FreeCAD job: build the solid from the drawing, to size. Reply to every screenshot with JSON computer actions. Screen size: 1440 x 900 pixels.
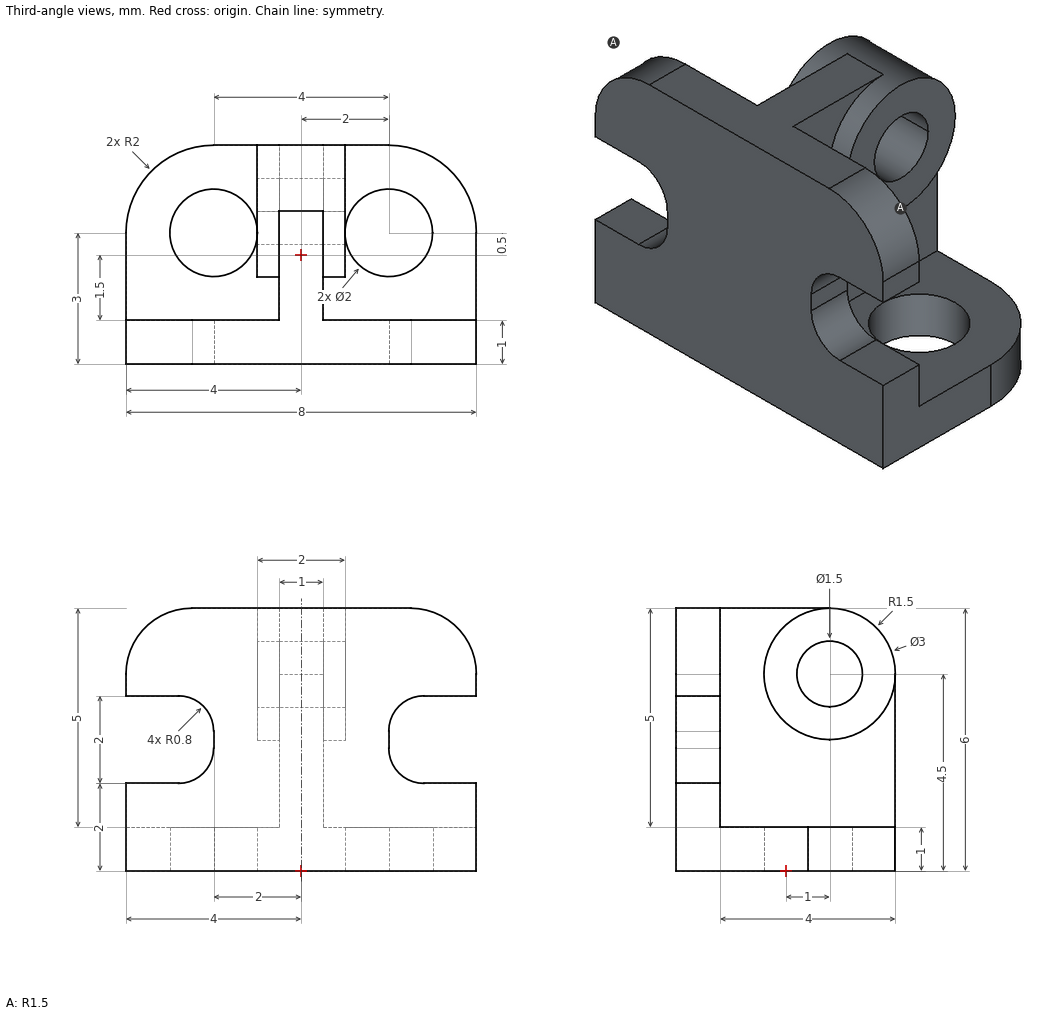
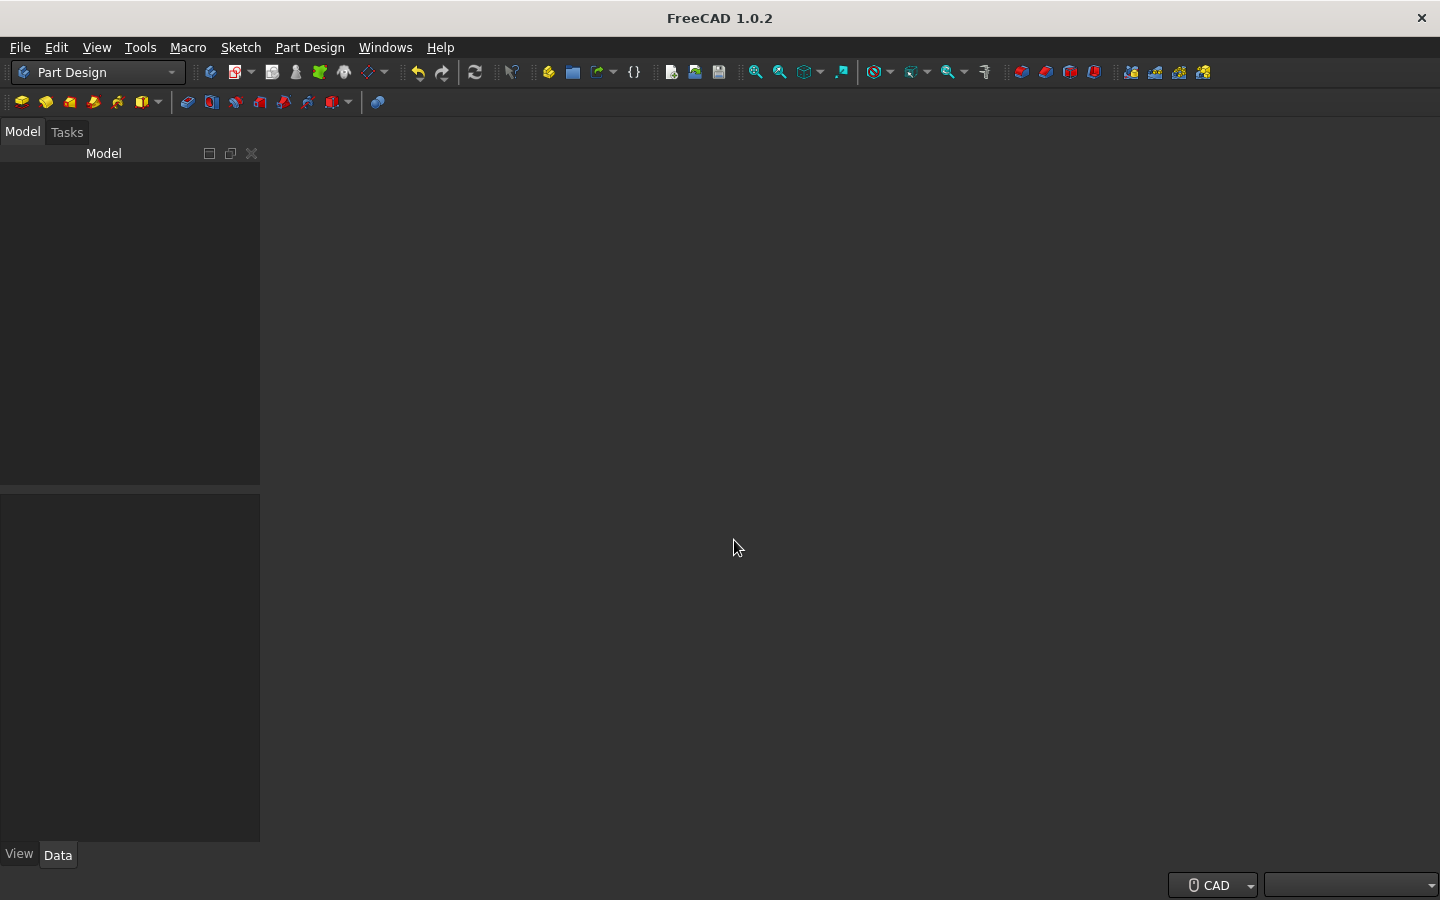
{"action": "left_click", "coordinate": [672, 72]}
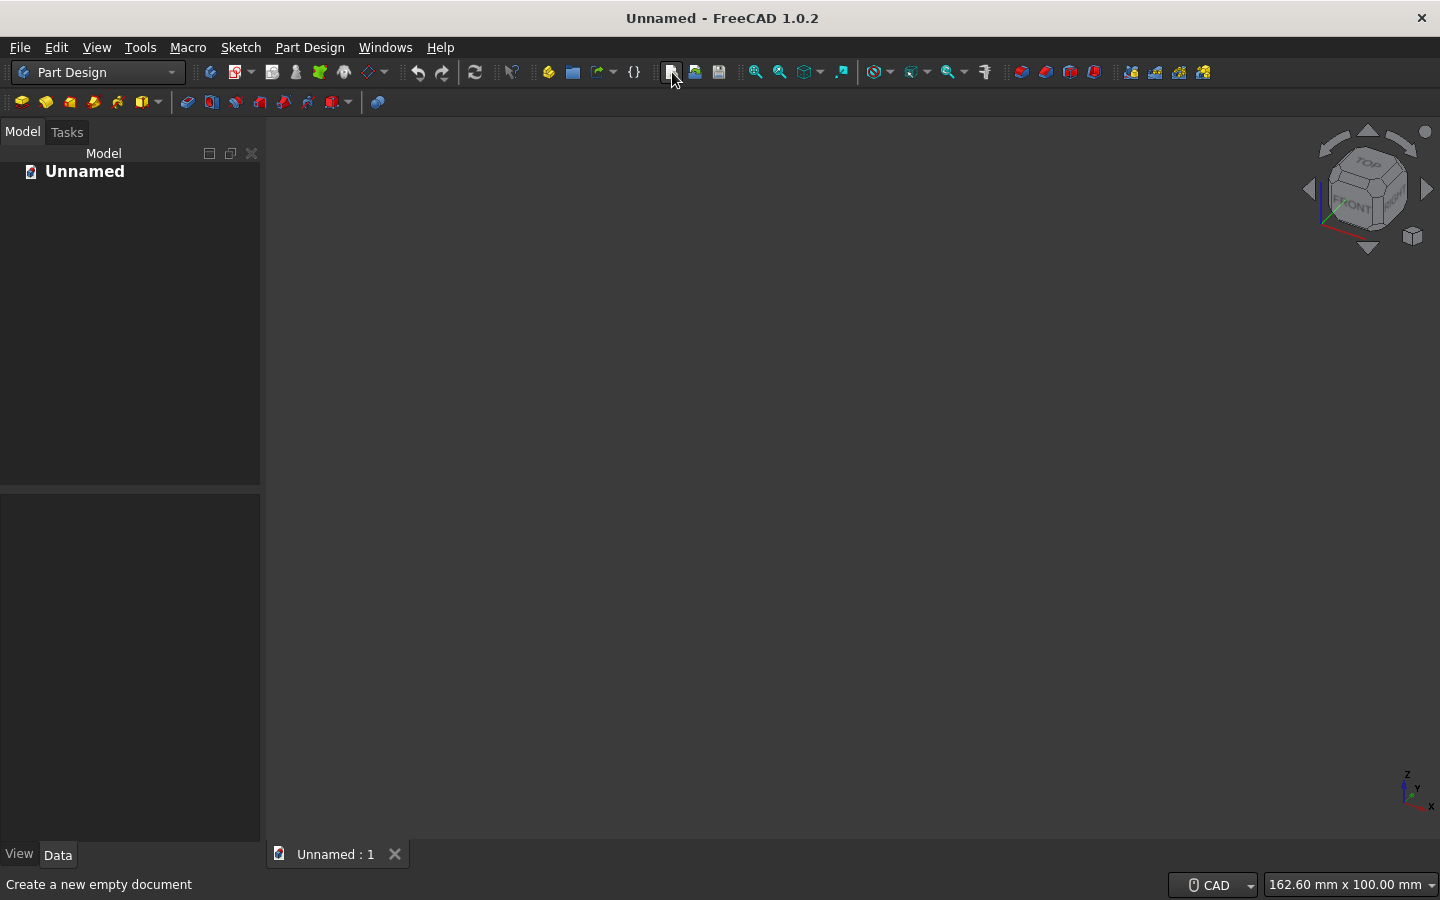
{"action": "left_click", "coordinate": [236, 72]}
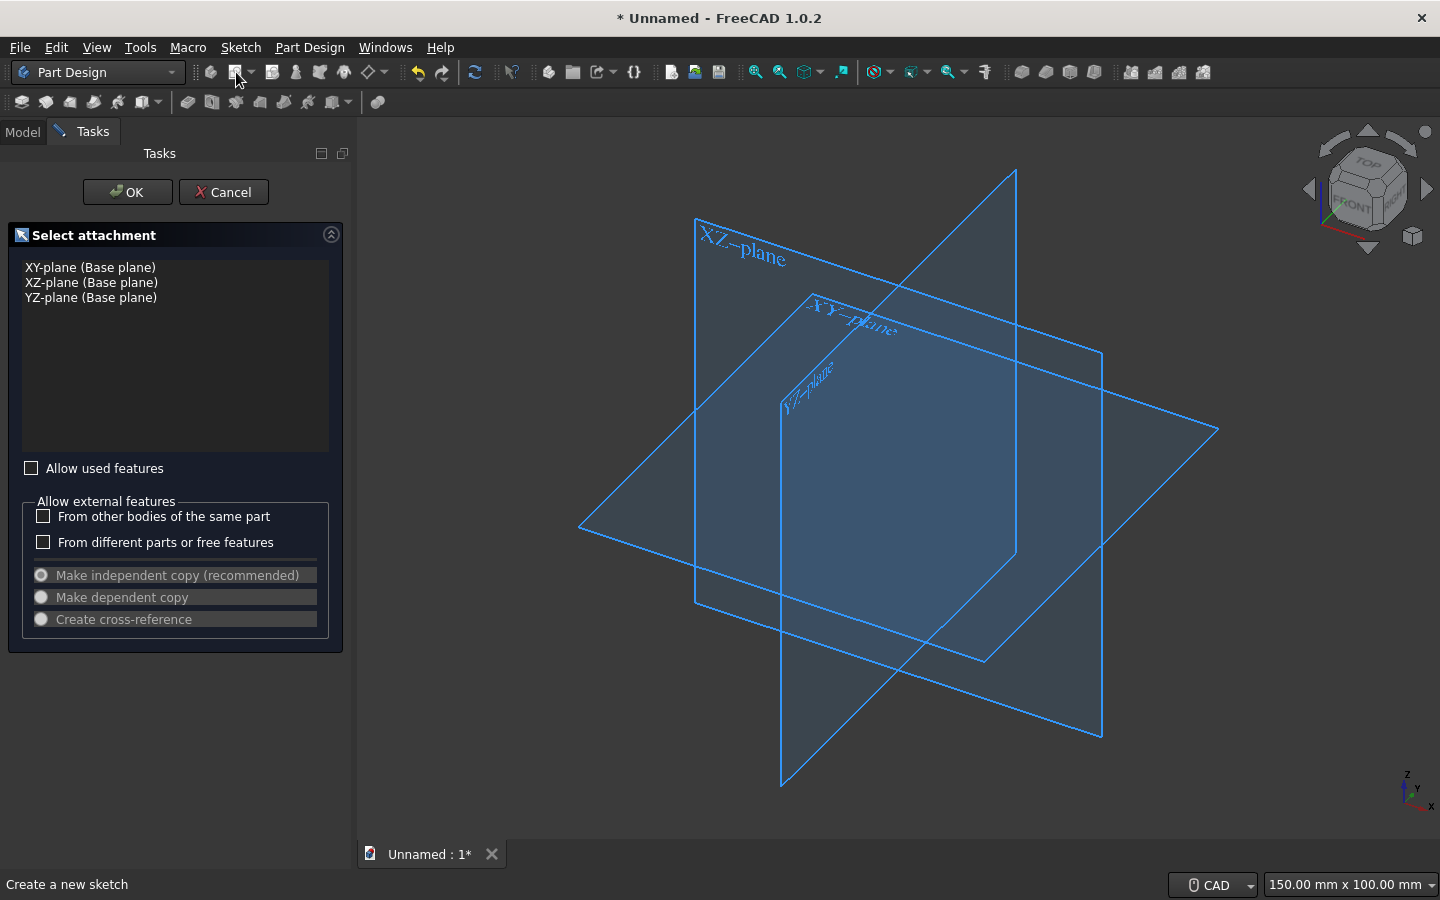
{"action": "left_click", "coordinate": [82, 268]}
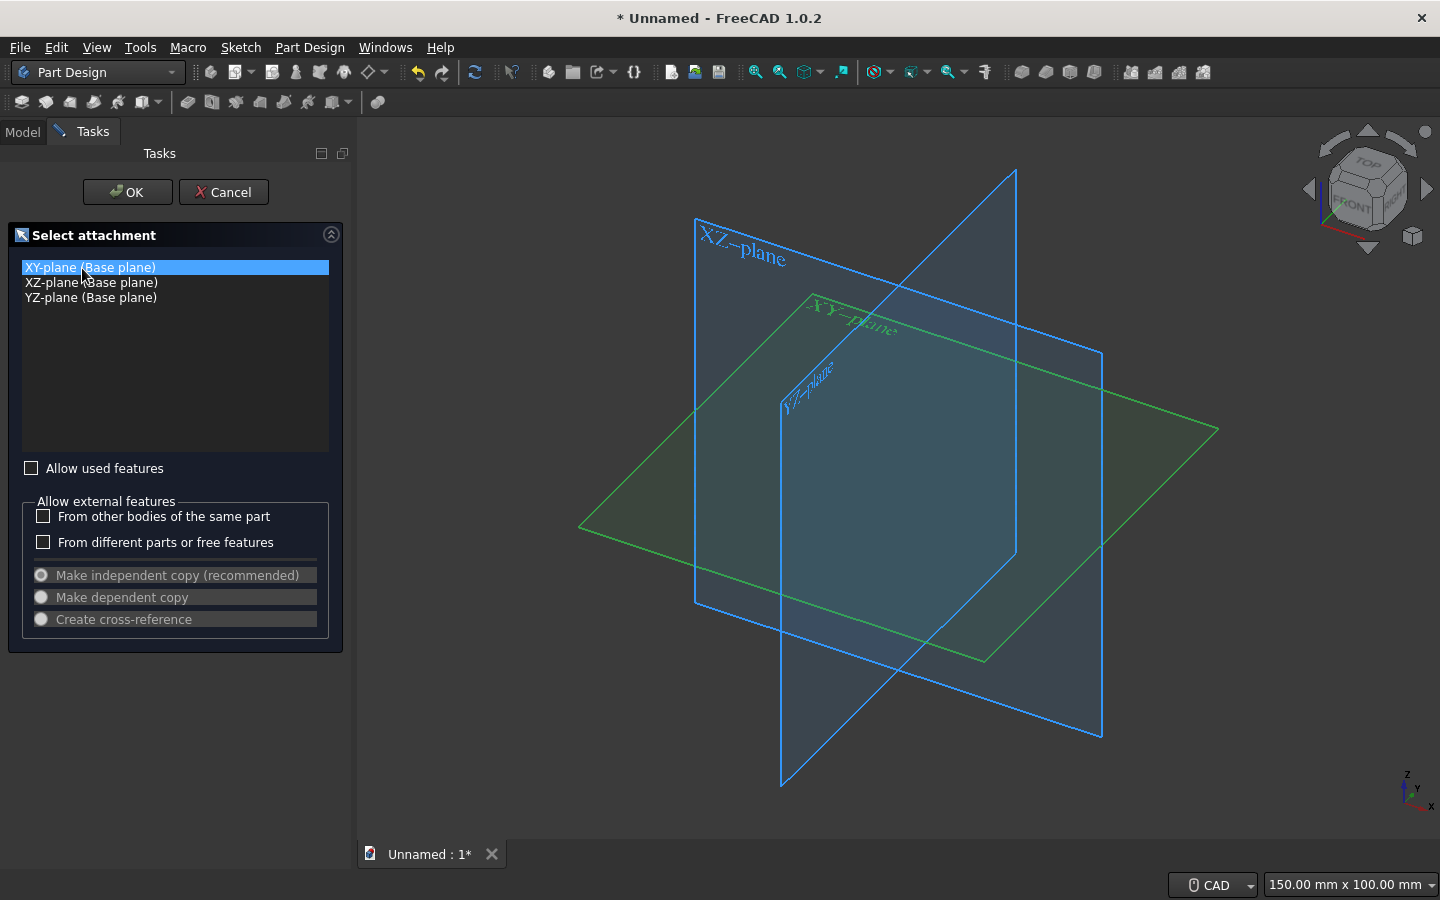
{"action": "left_click", "coordinate": [128, 192]}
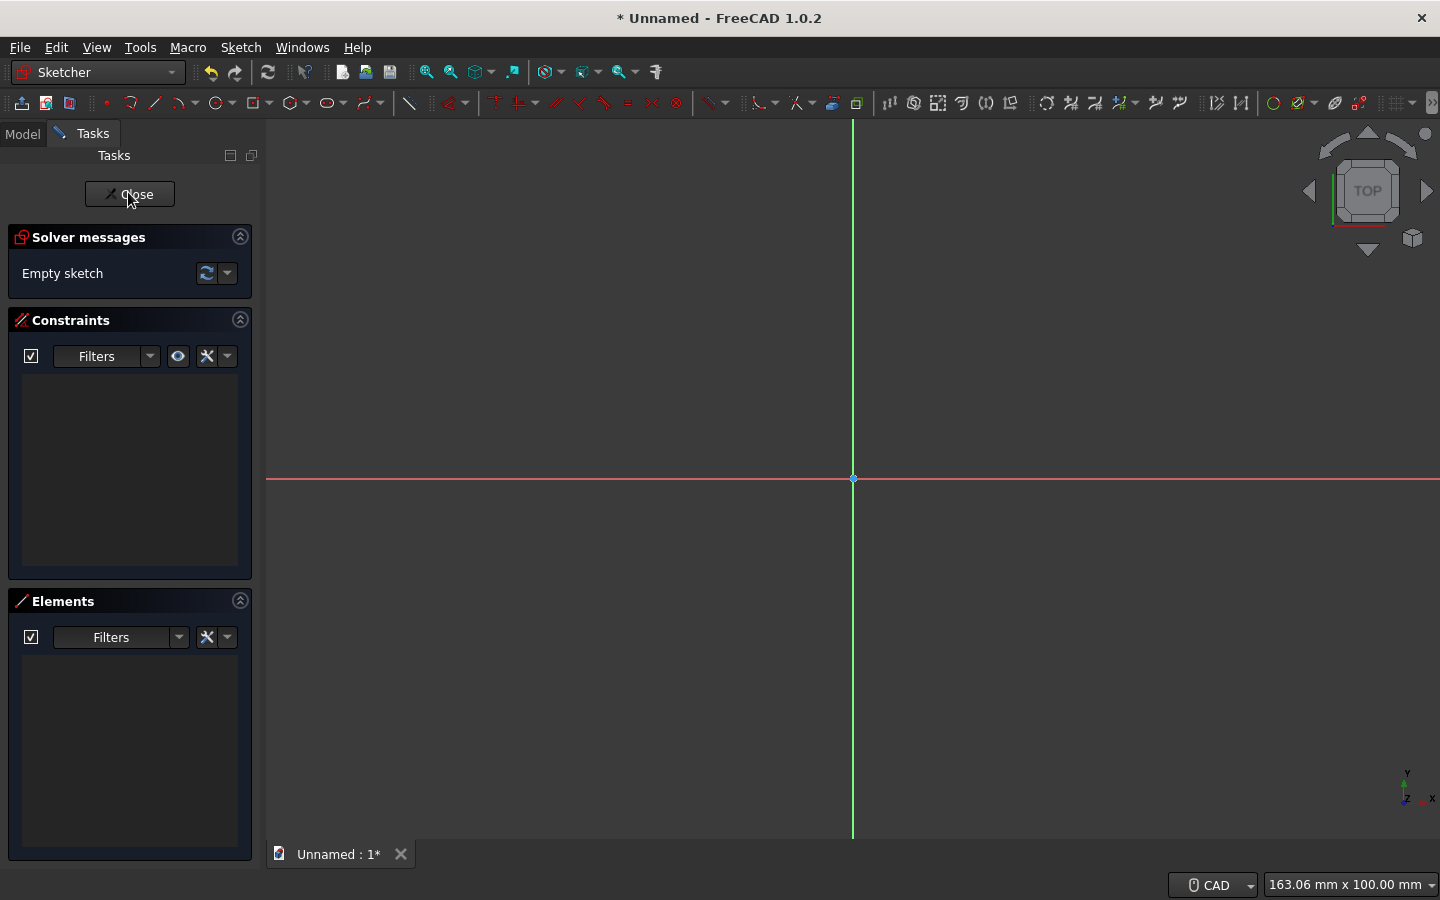
{"action": "scroll", "coordinate": [860, 479], "scroll_direction": "up", "scroll_amount": 12}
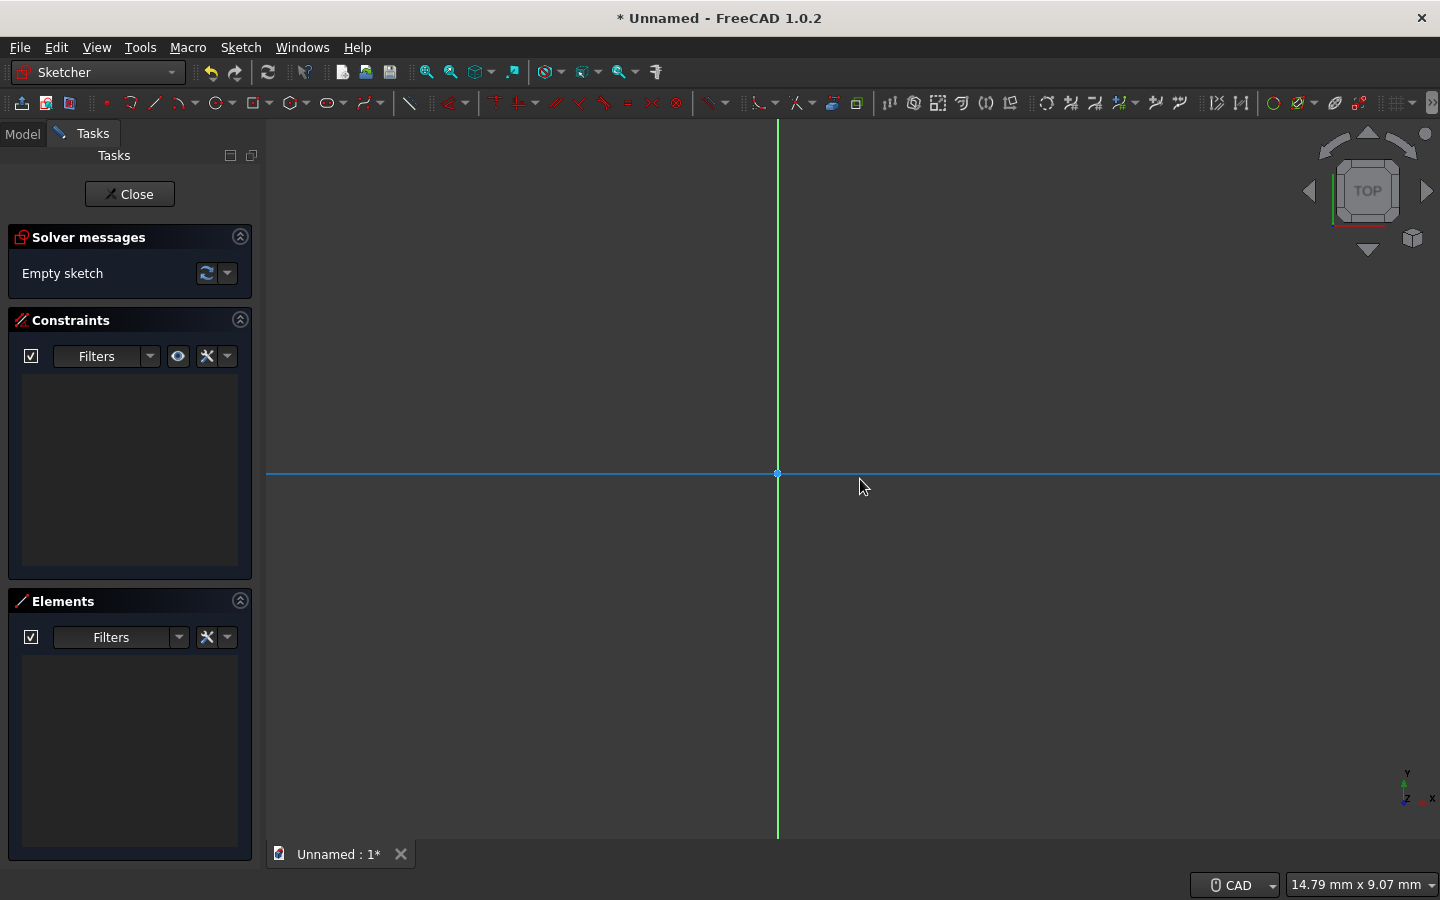
{"action": "key", "text": "g l"}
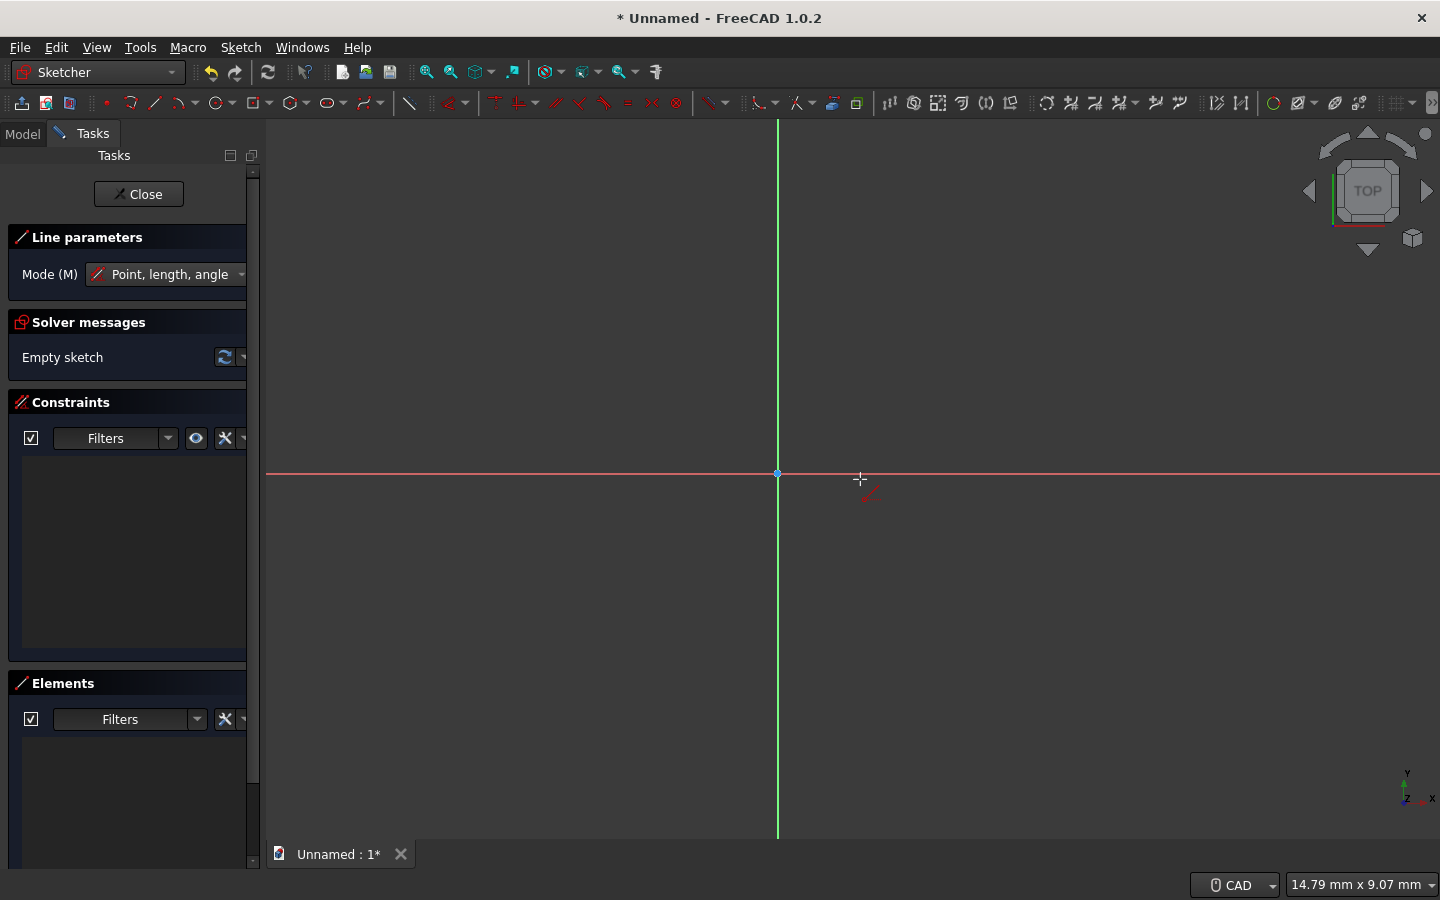
{"action": "left_click", "coordinate": [936, 276]}
{"action": "left_click", "coordinate": [619, 276]}